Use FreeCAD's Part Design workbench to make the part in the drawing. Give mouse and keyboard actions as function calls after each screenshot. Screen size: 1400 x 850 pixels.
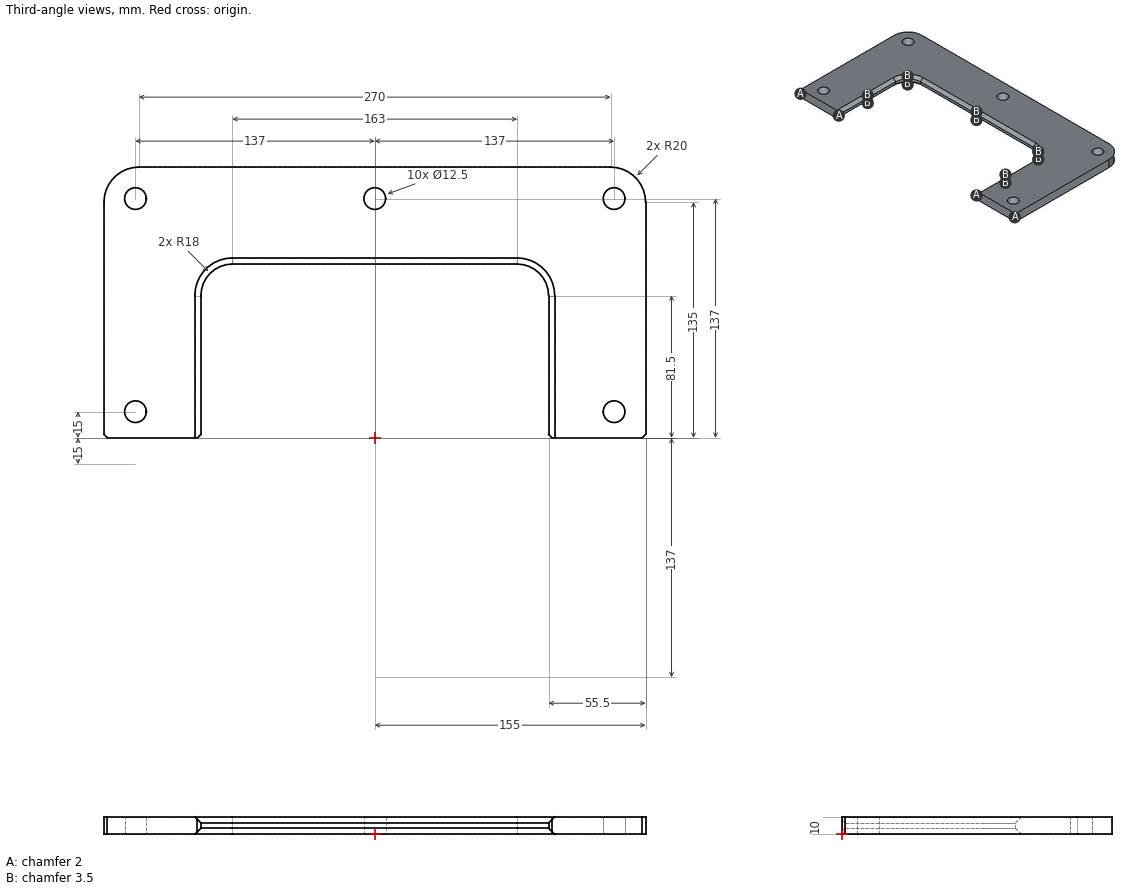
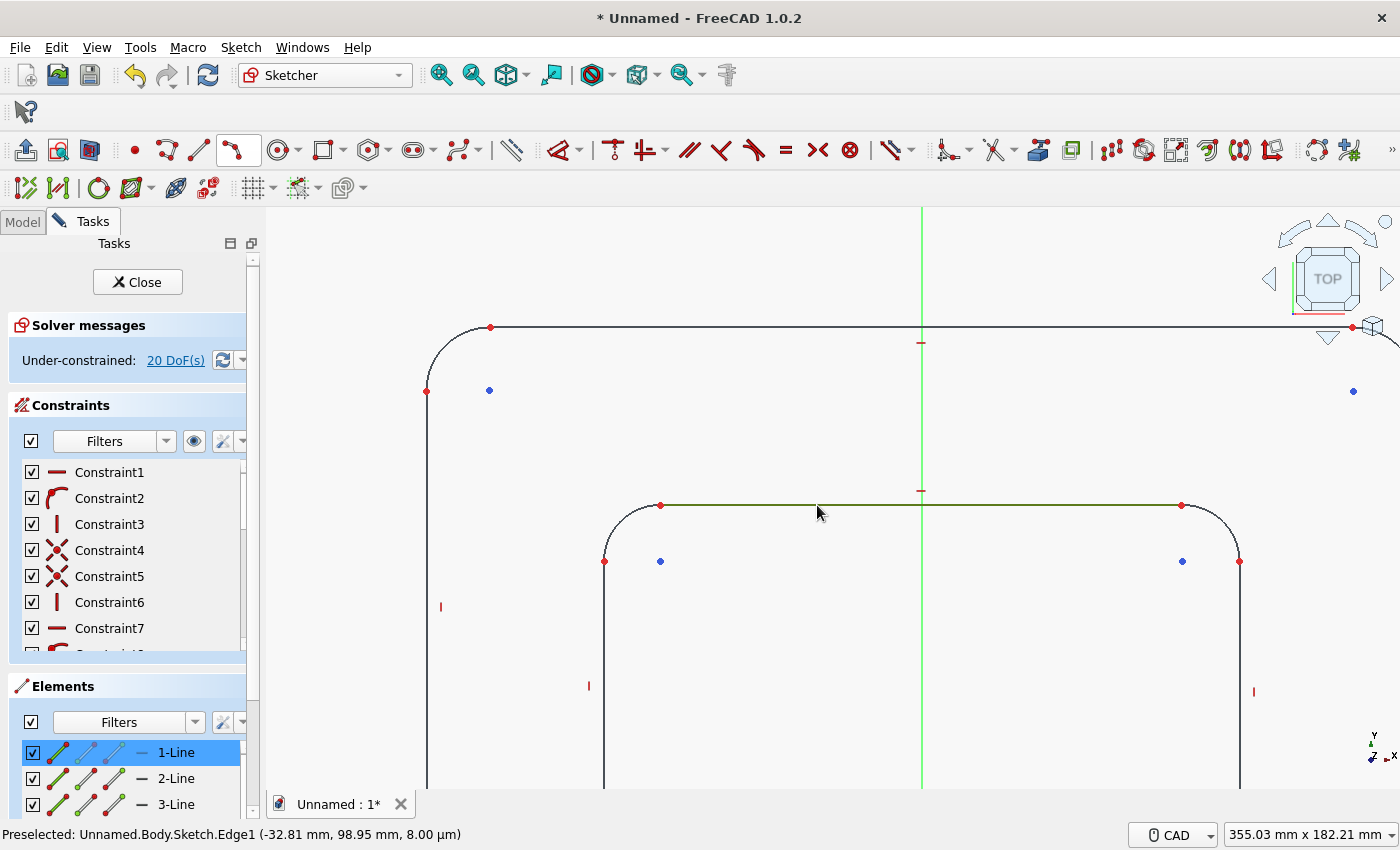
click(1233, 536)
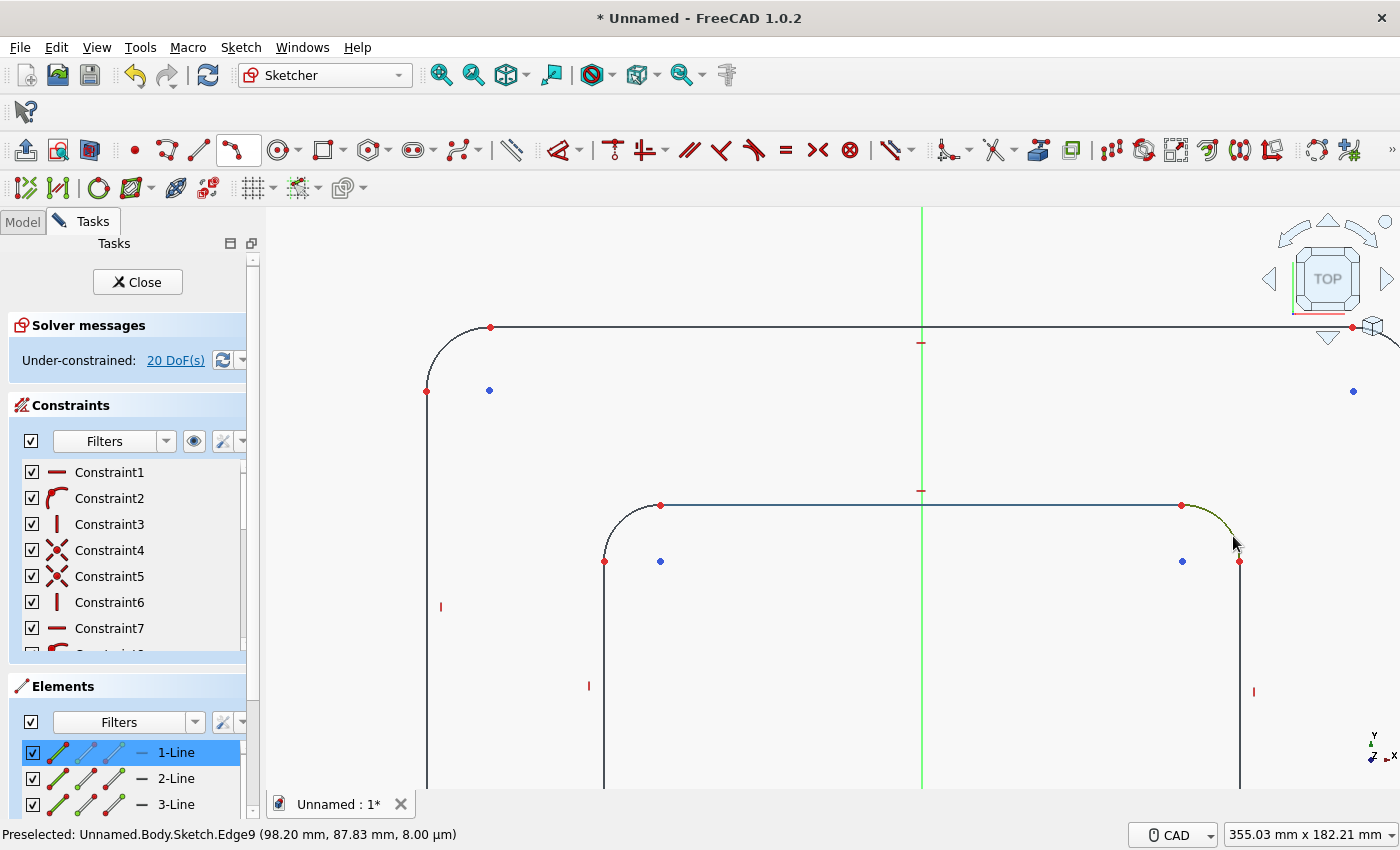
key(t)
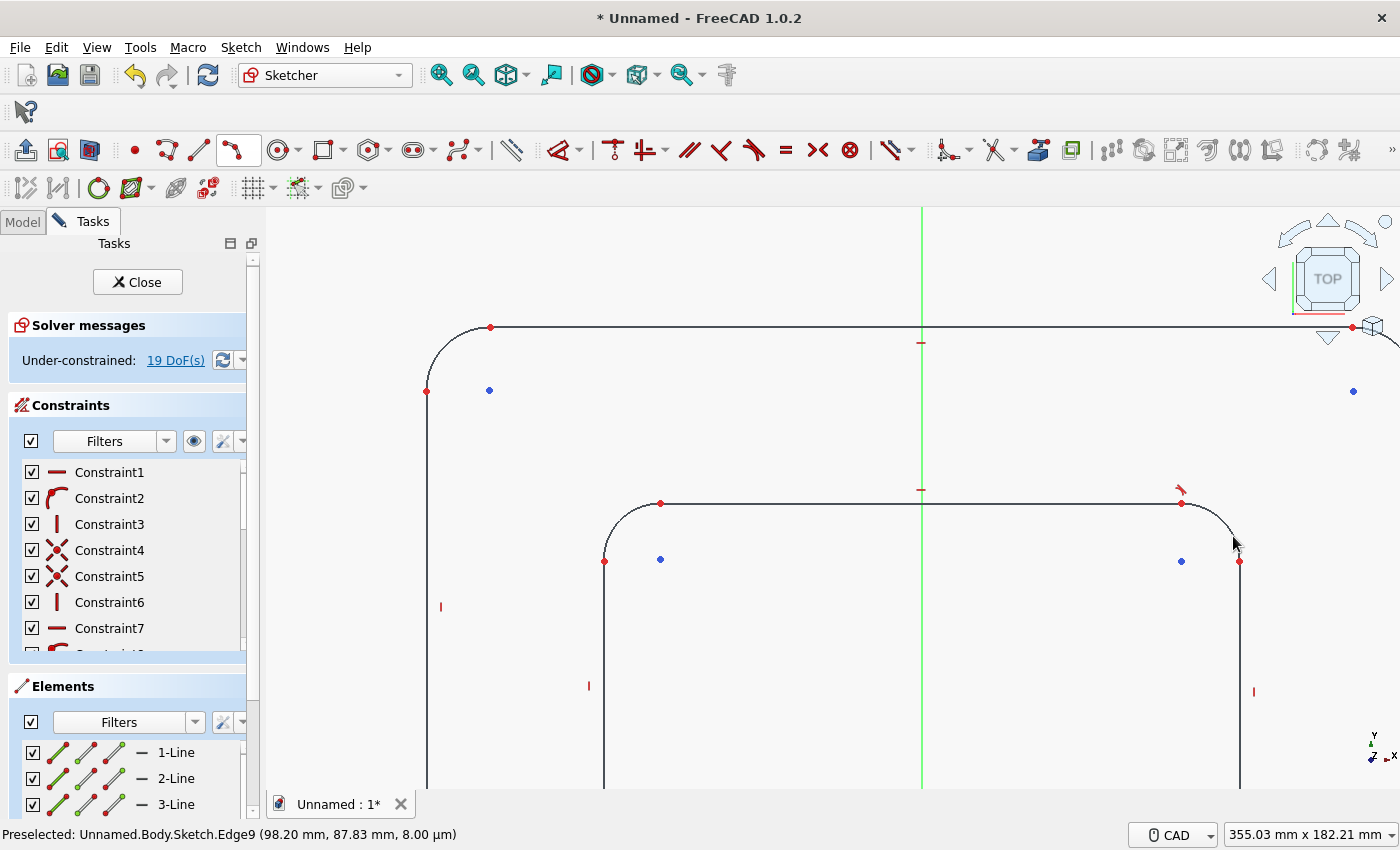
click(817, 504)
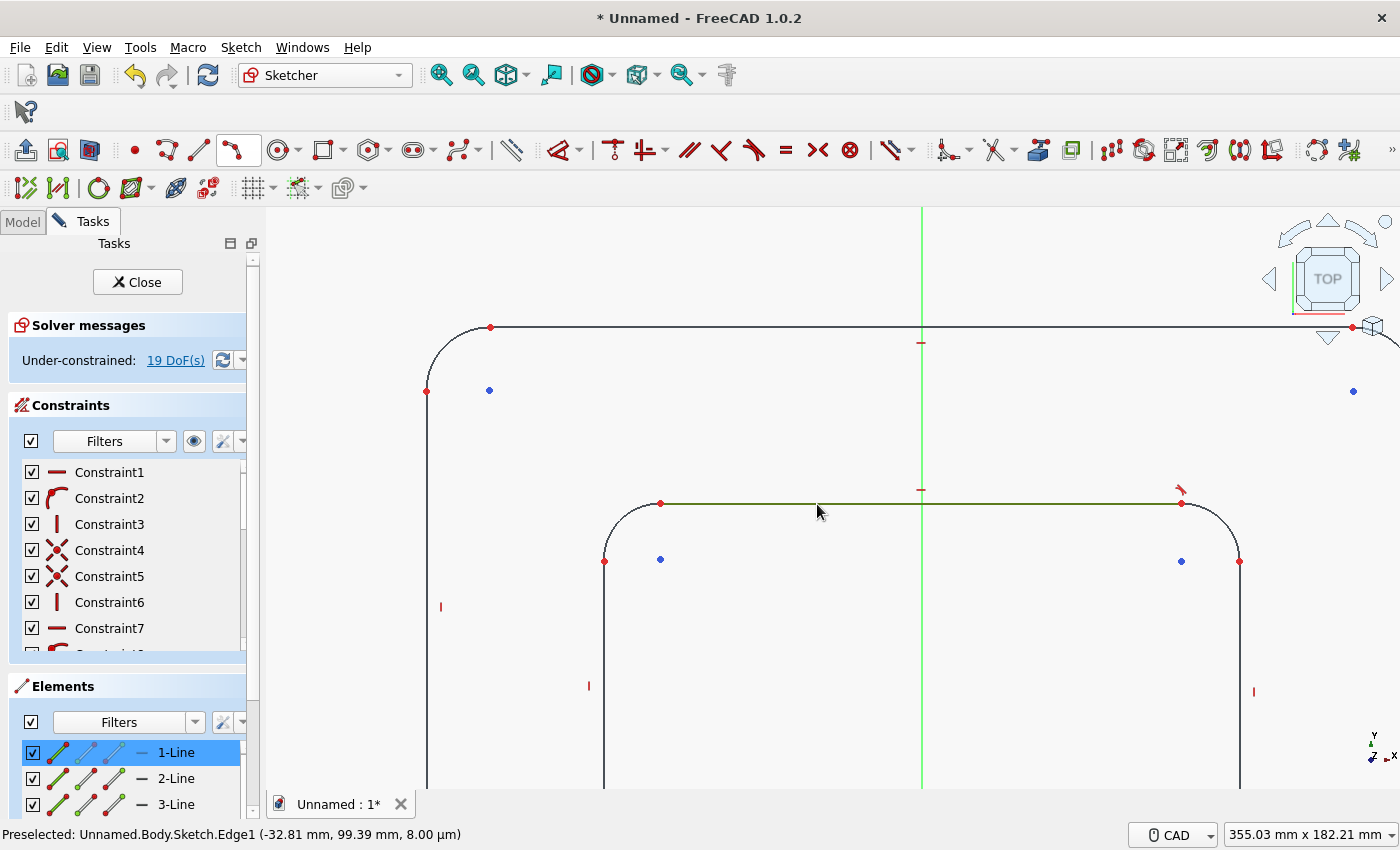
click(635, 510)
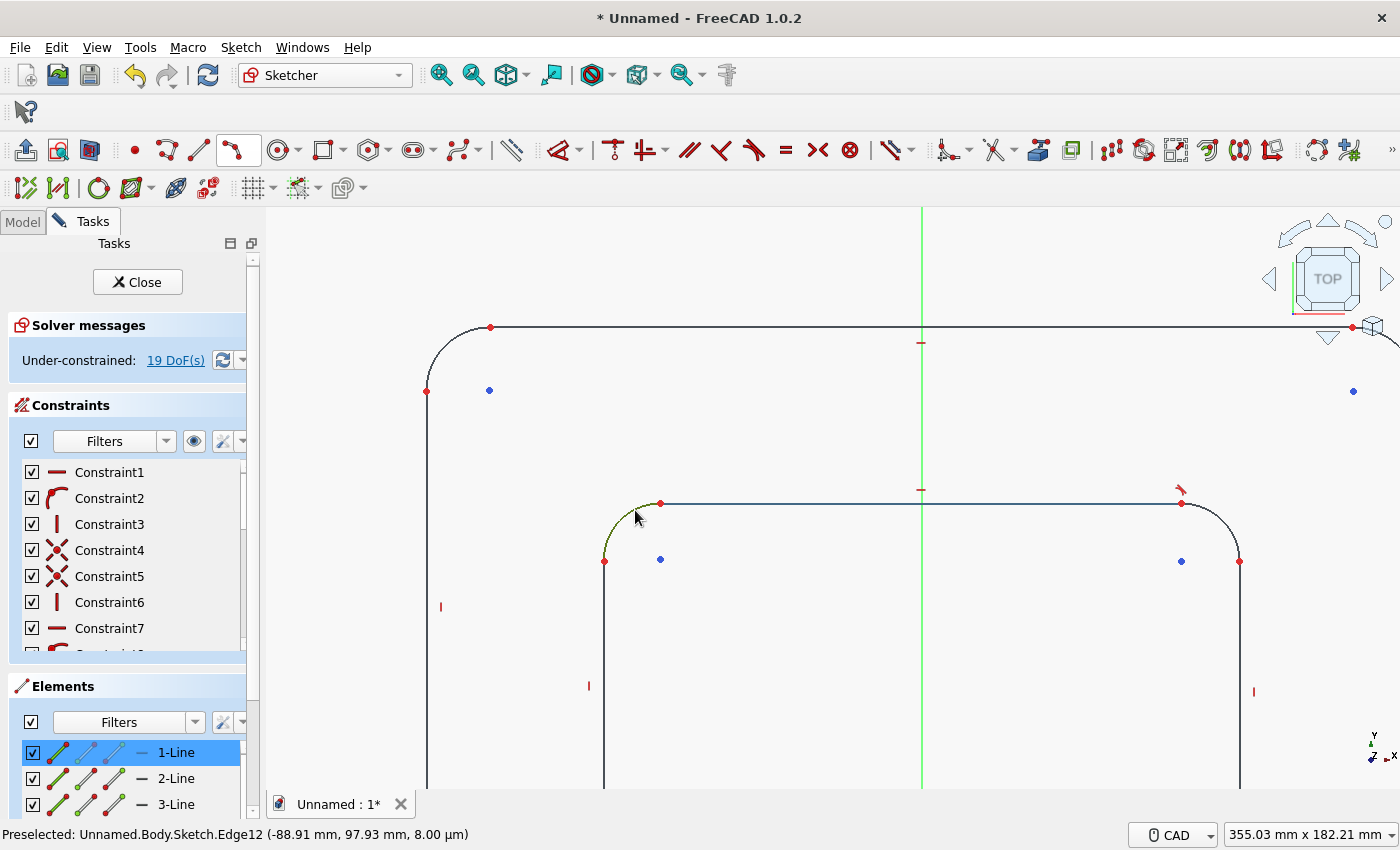
click(754, 150)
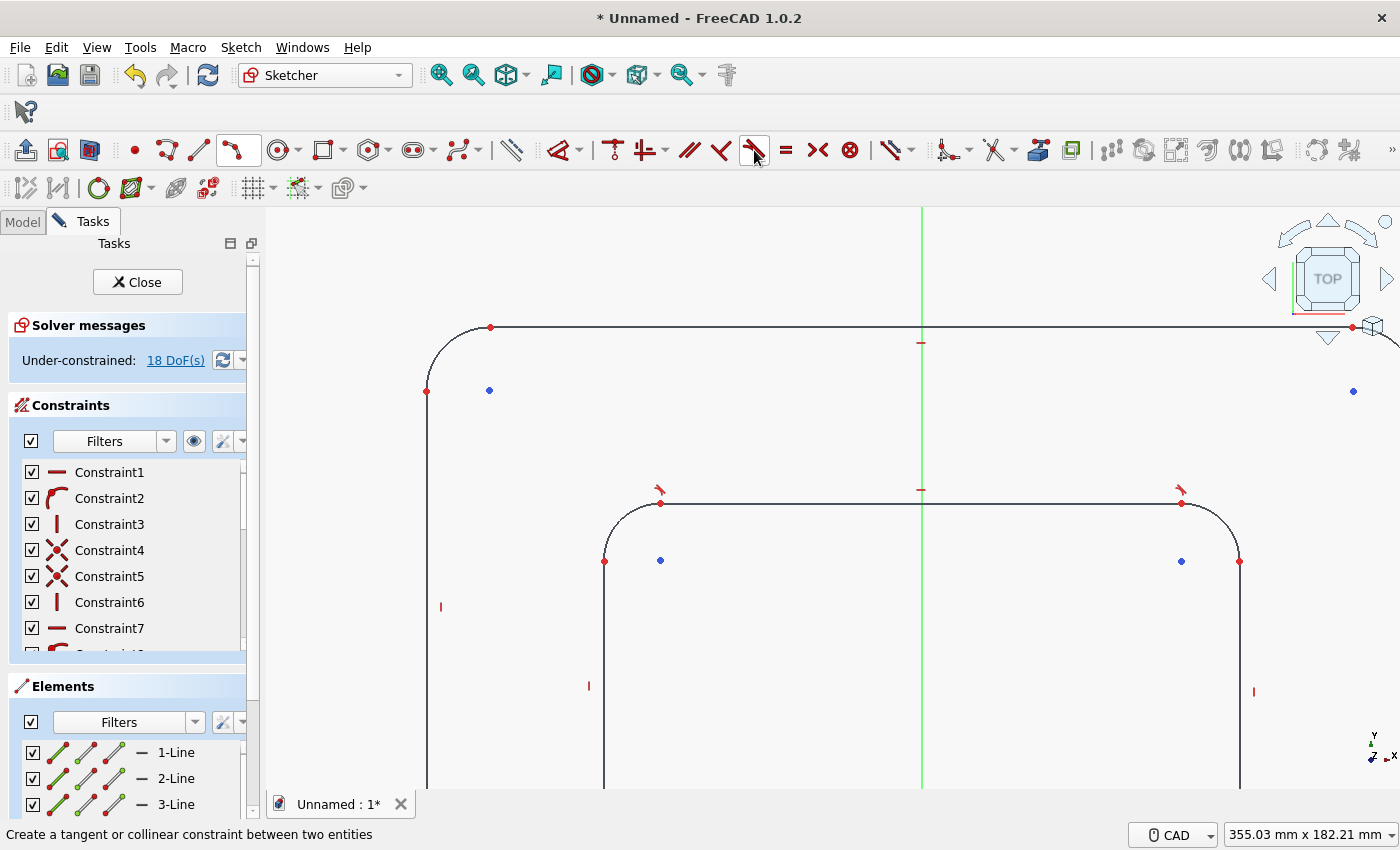
scroll(445, 344, down, 2)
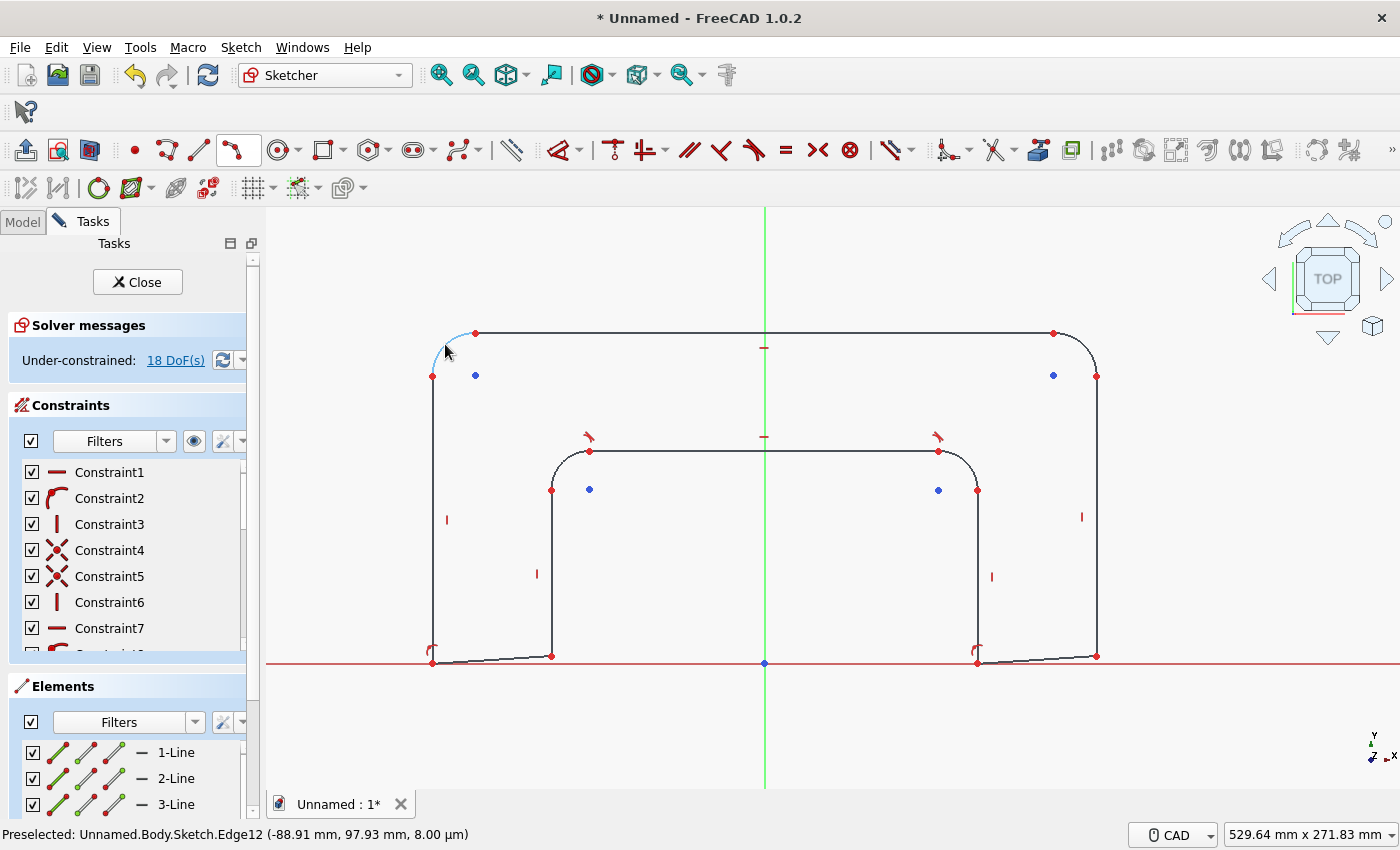
click(978, 542)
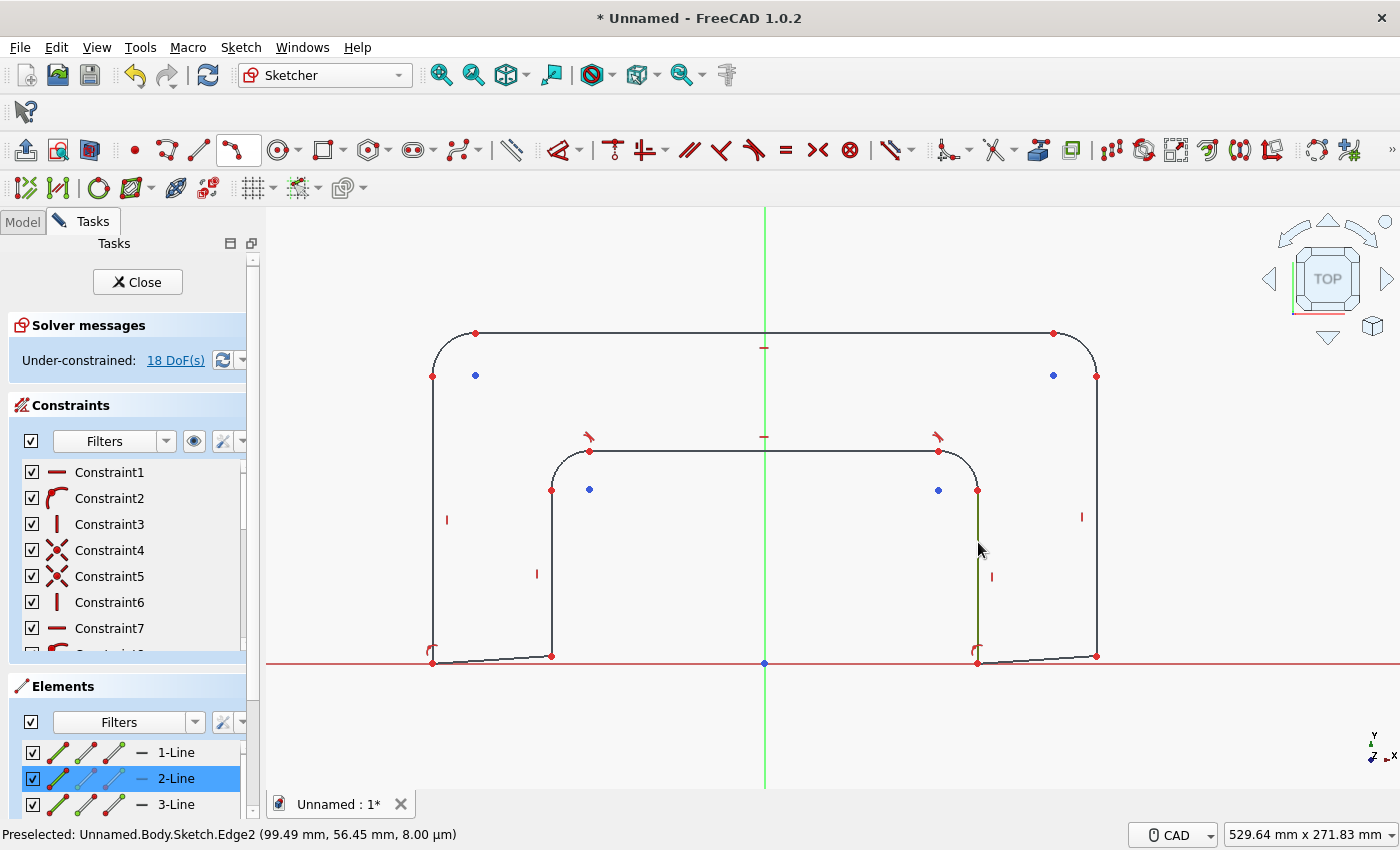
click(973, 472)